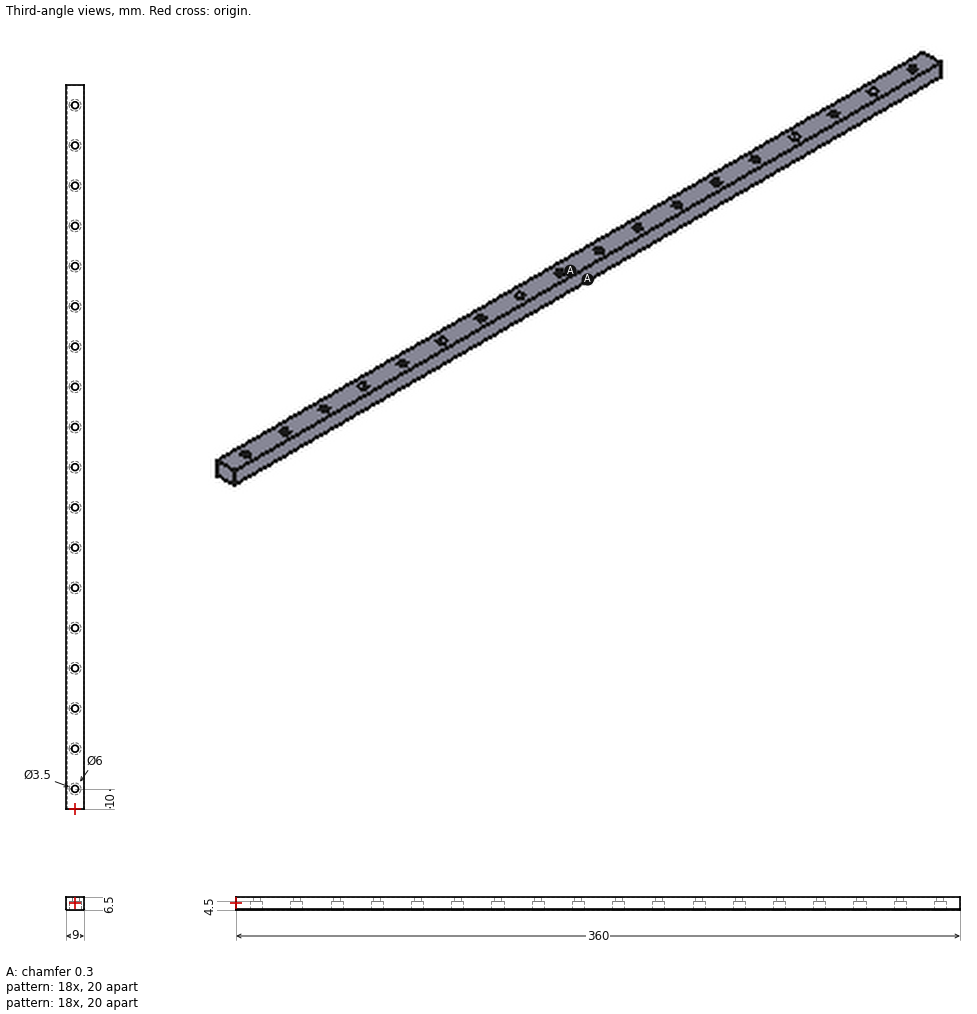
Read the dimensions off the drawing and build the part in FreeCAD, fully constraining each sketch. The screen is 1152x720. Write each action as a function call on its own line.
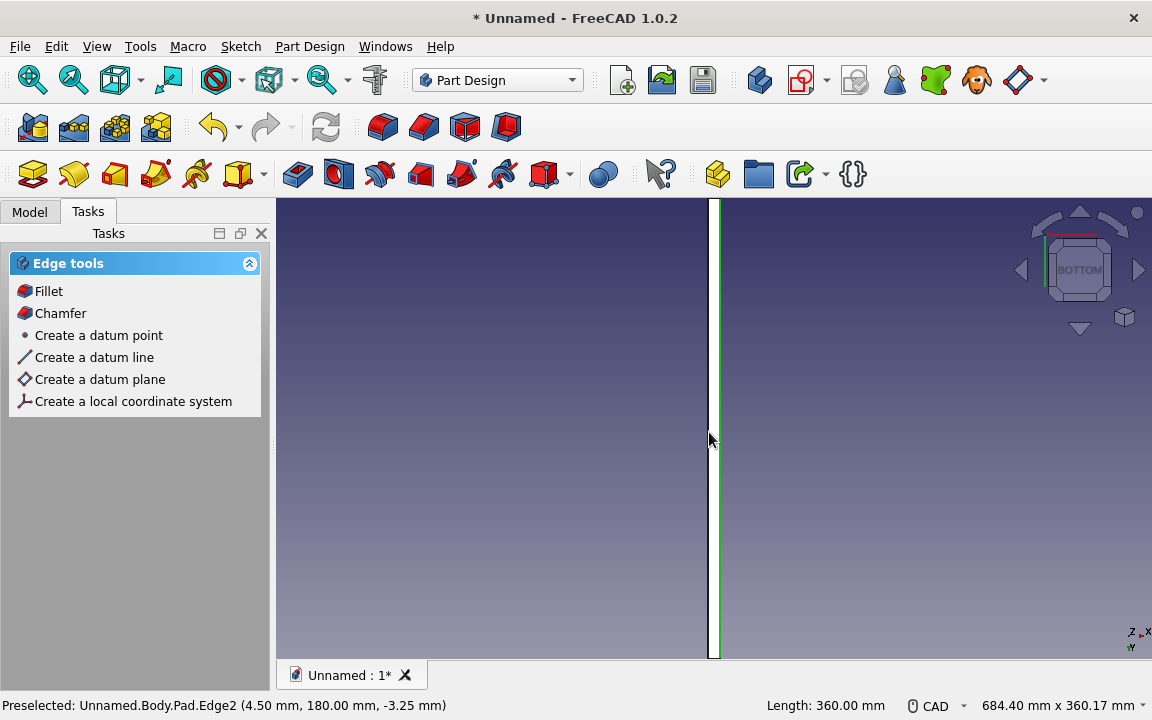
click(708, 427, ctrl)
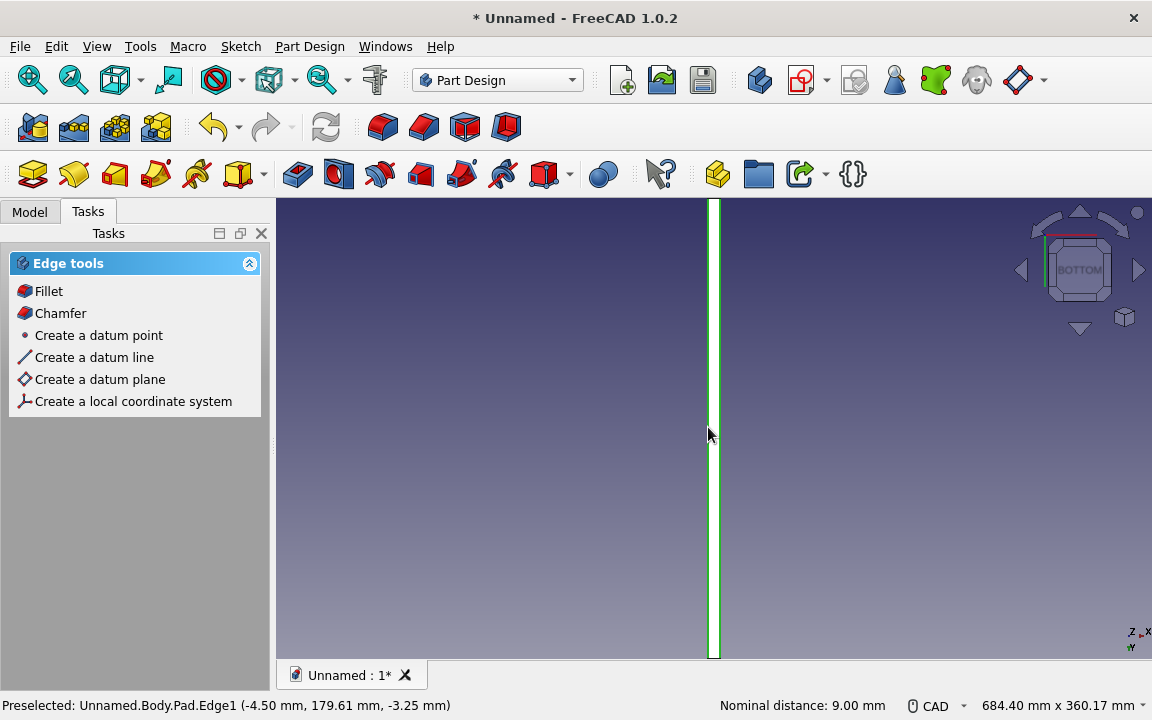
click(424, 128)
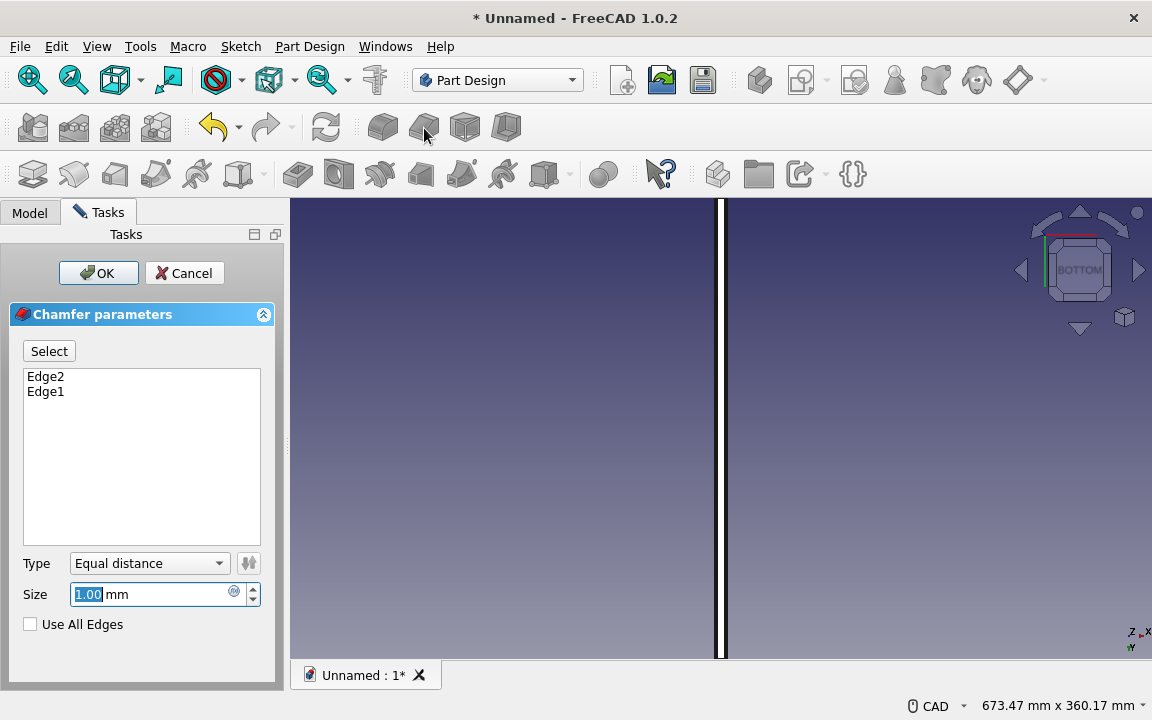
text(0.3)
key(Tab)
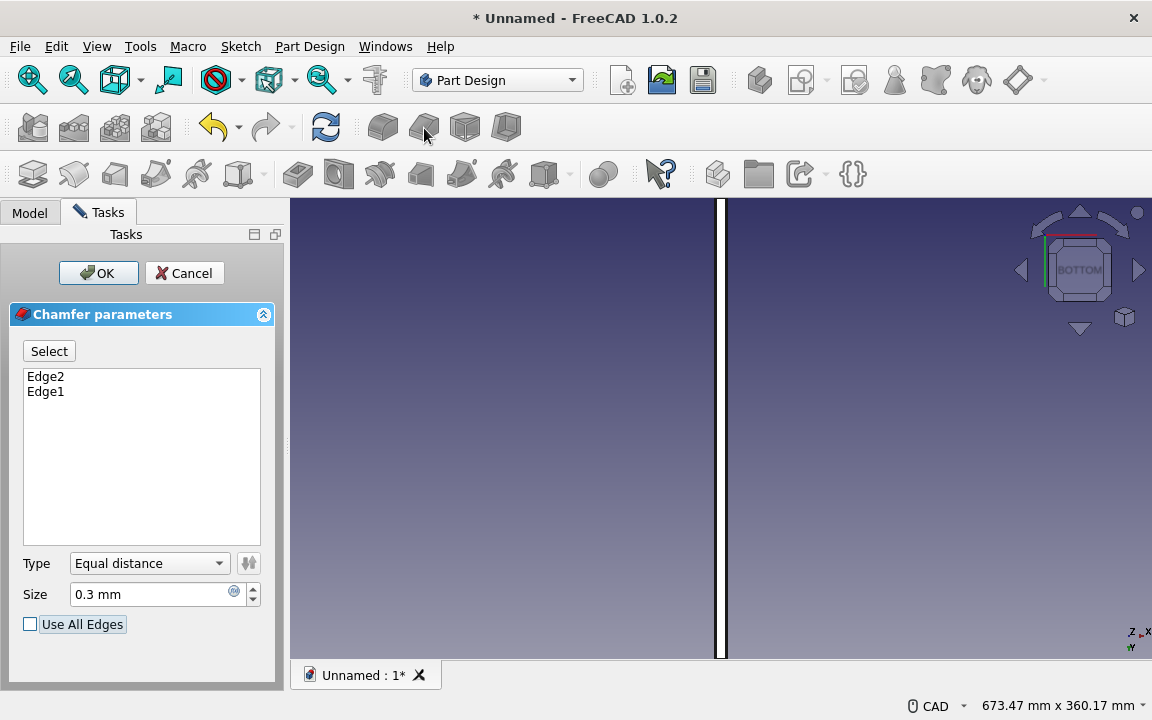
click(99, 273)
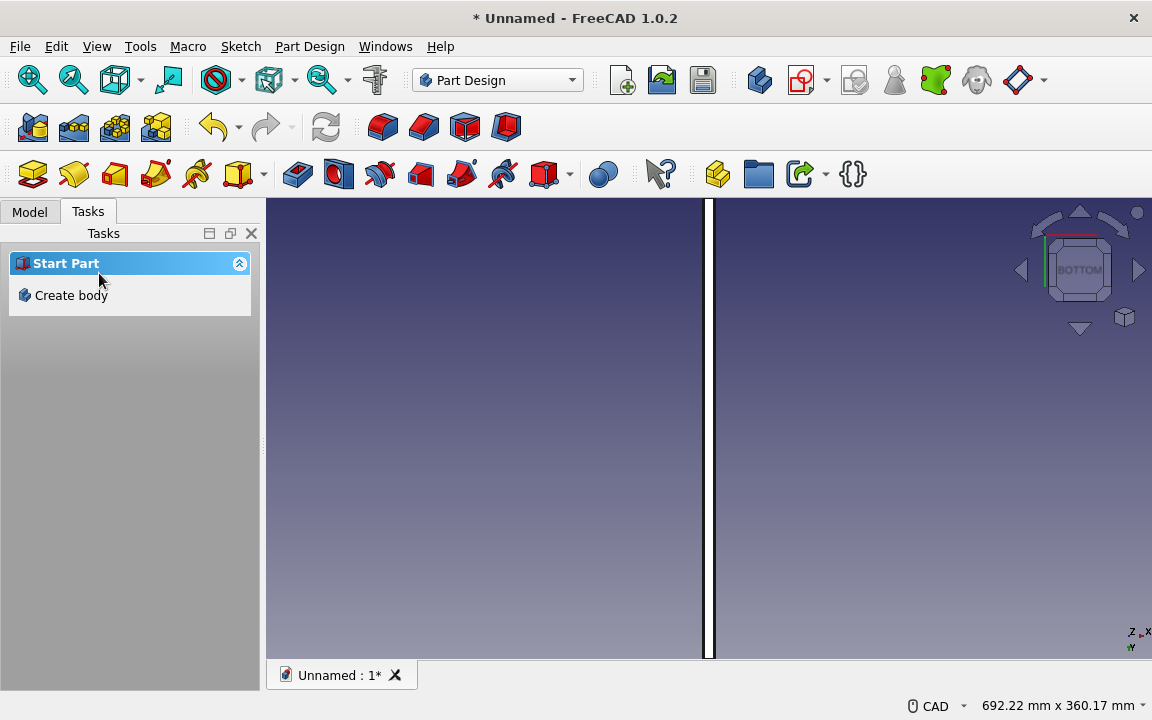
key(v)
key(f)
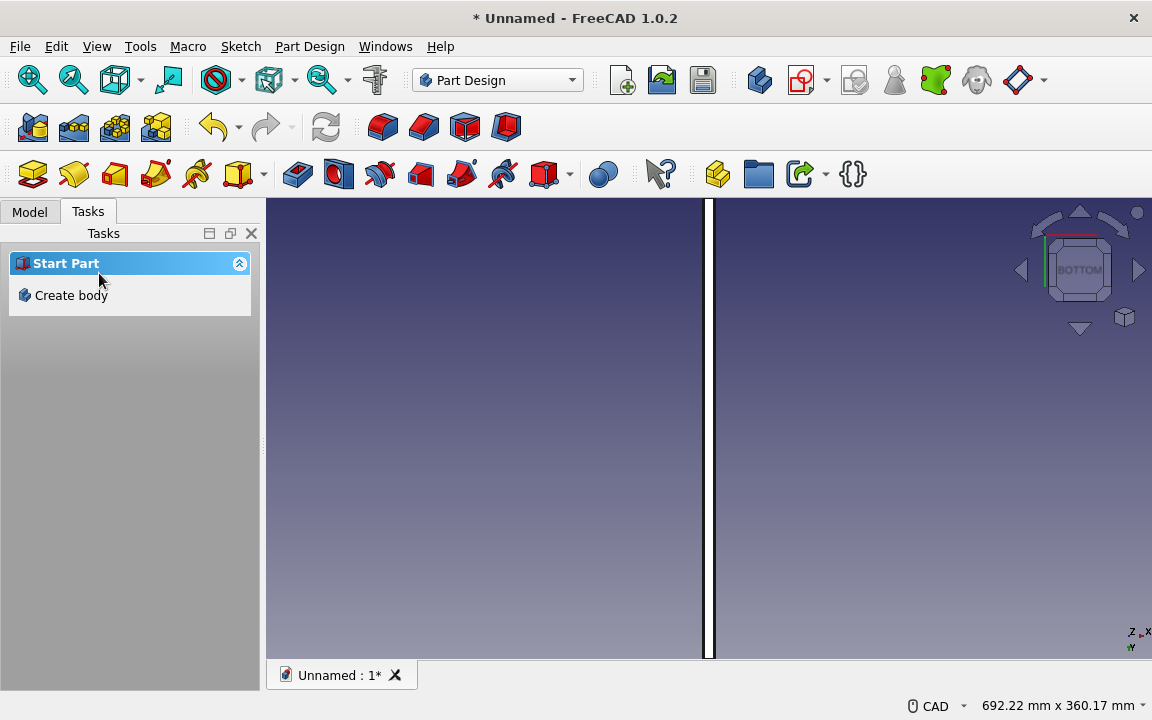
scroll(709, 625, up, 5)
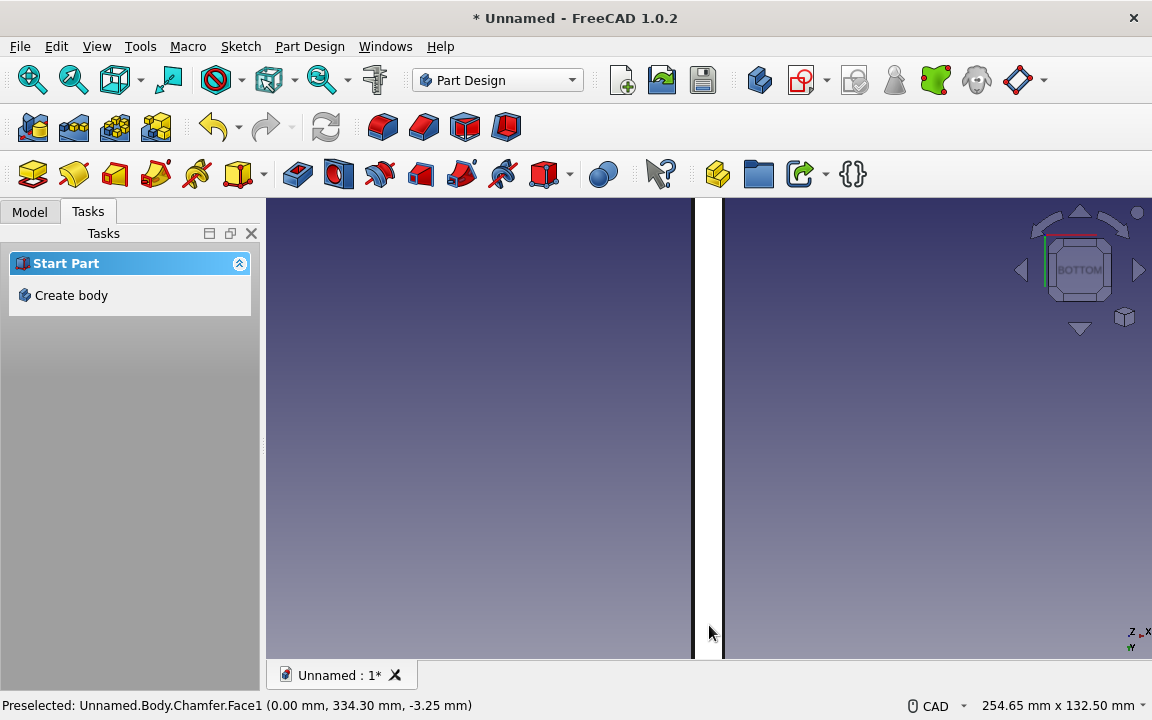
click(708, 625)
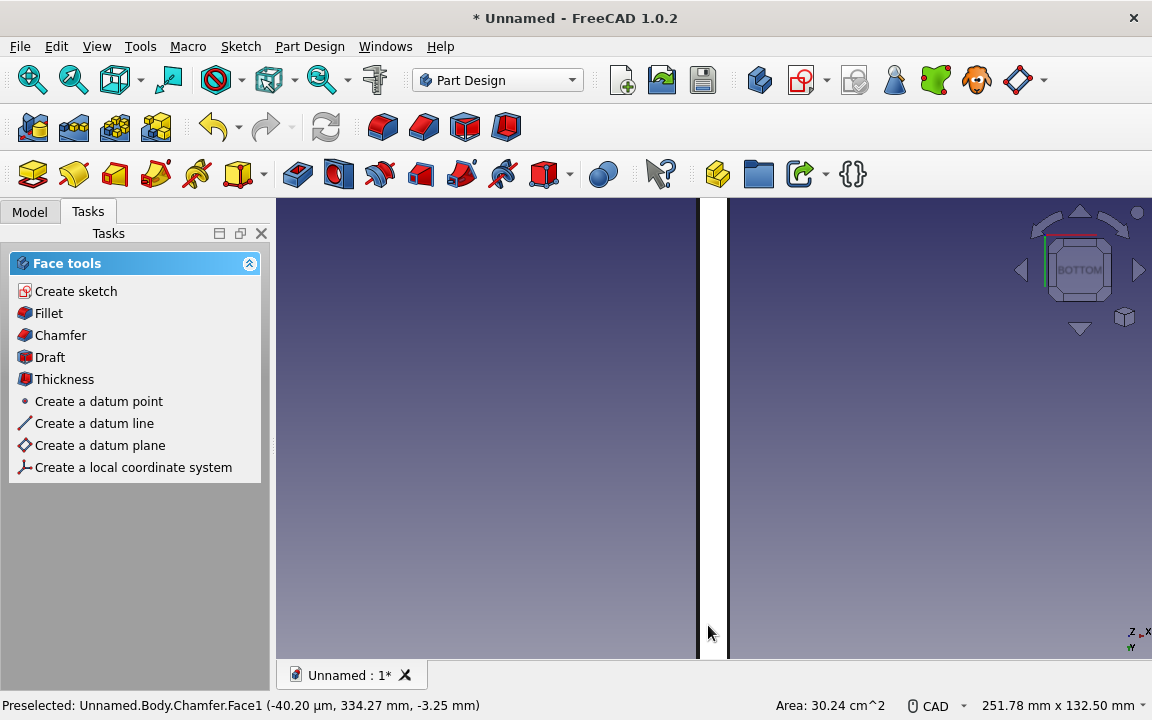
click(800, 80)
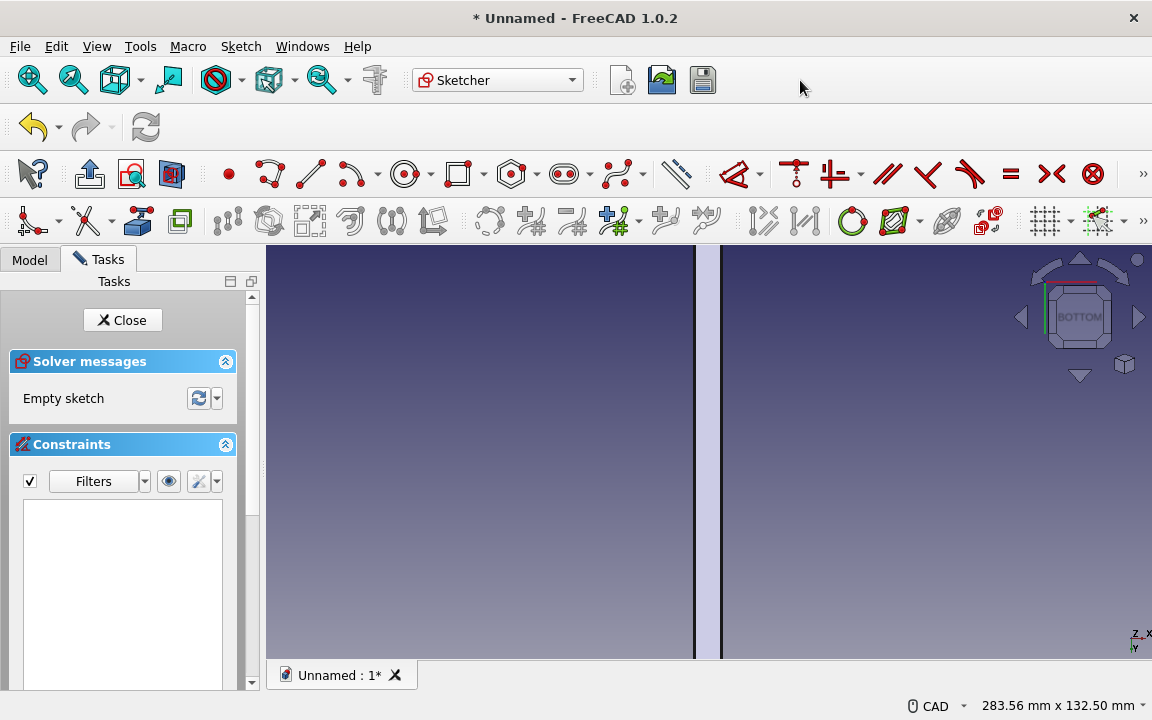
scroll(640, 452, down, 5)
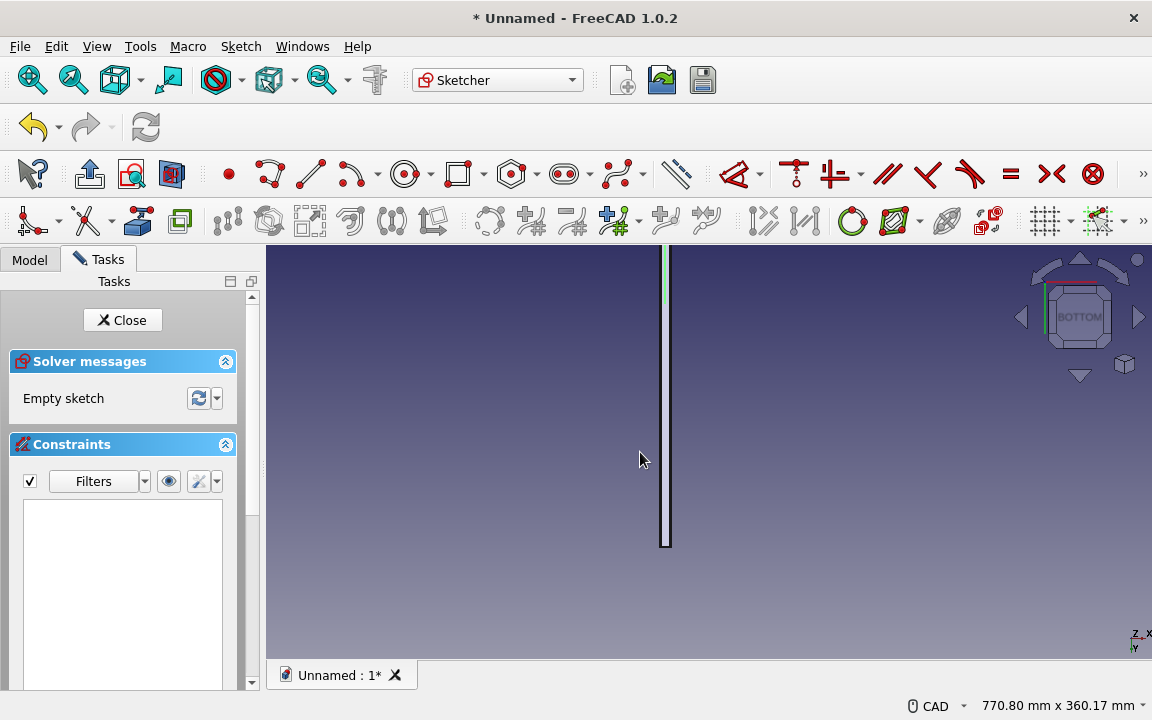
scroll(640, 452, down, 5)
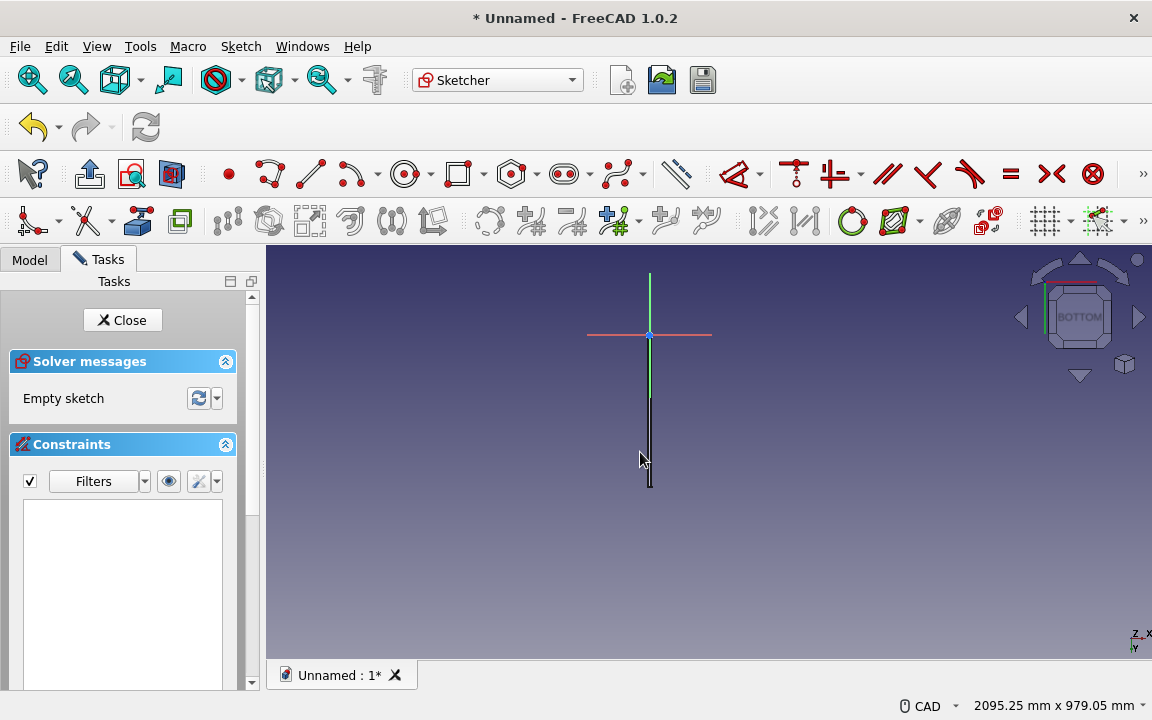
scroll(650, 333, up, 15)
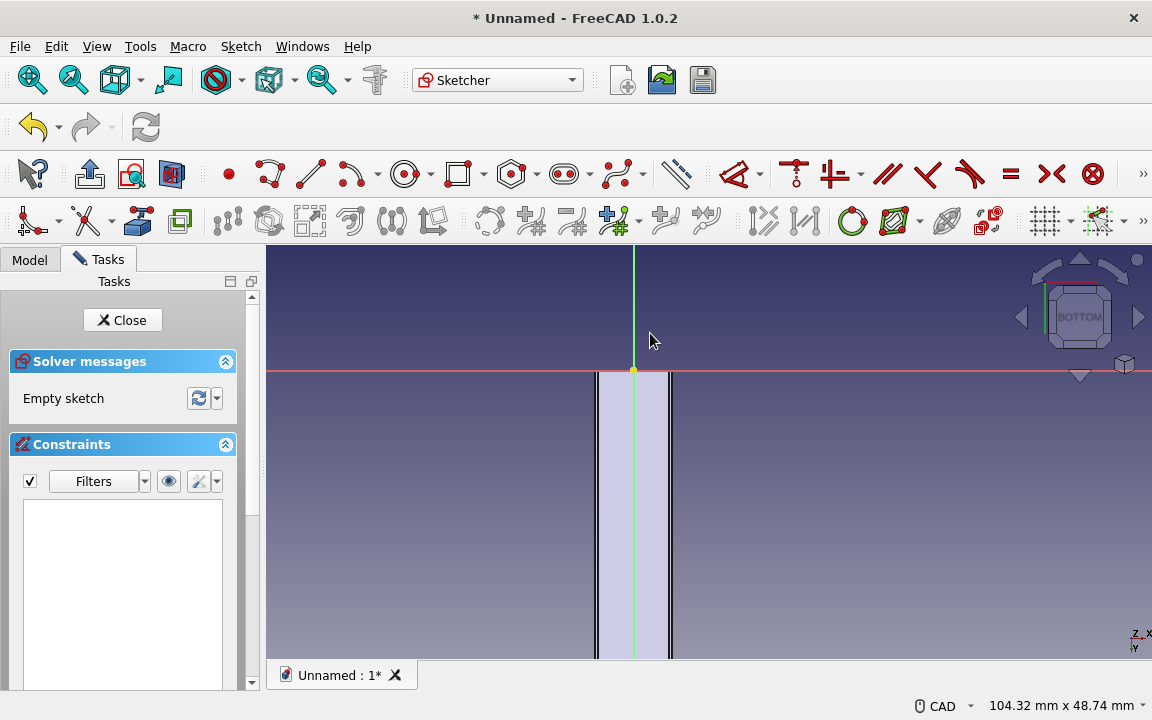
scroll(633, 456, up, 11)